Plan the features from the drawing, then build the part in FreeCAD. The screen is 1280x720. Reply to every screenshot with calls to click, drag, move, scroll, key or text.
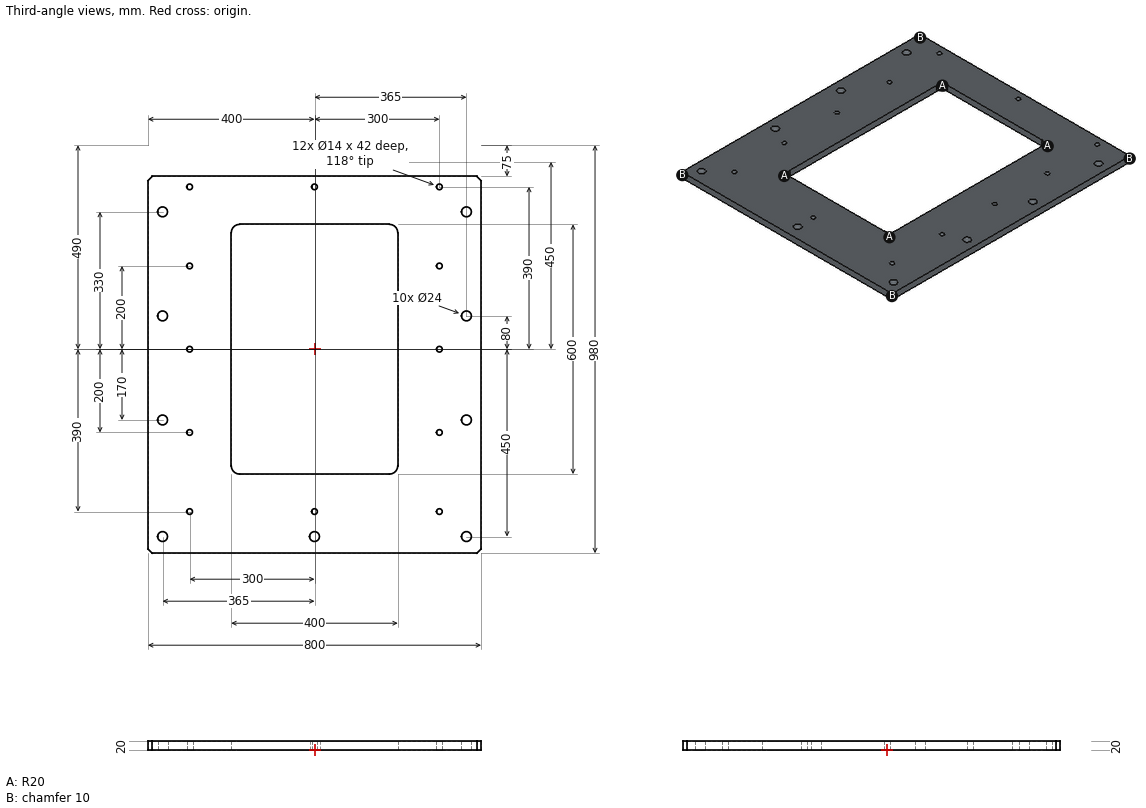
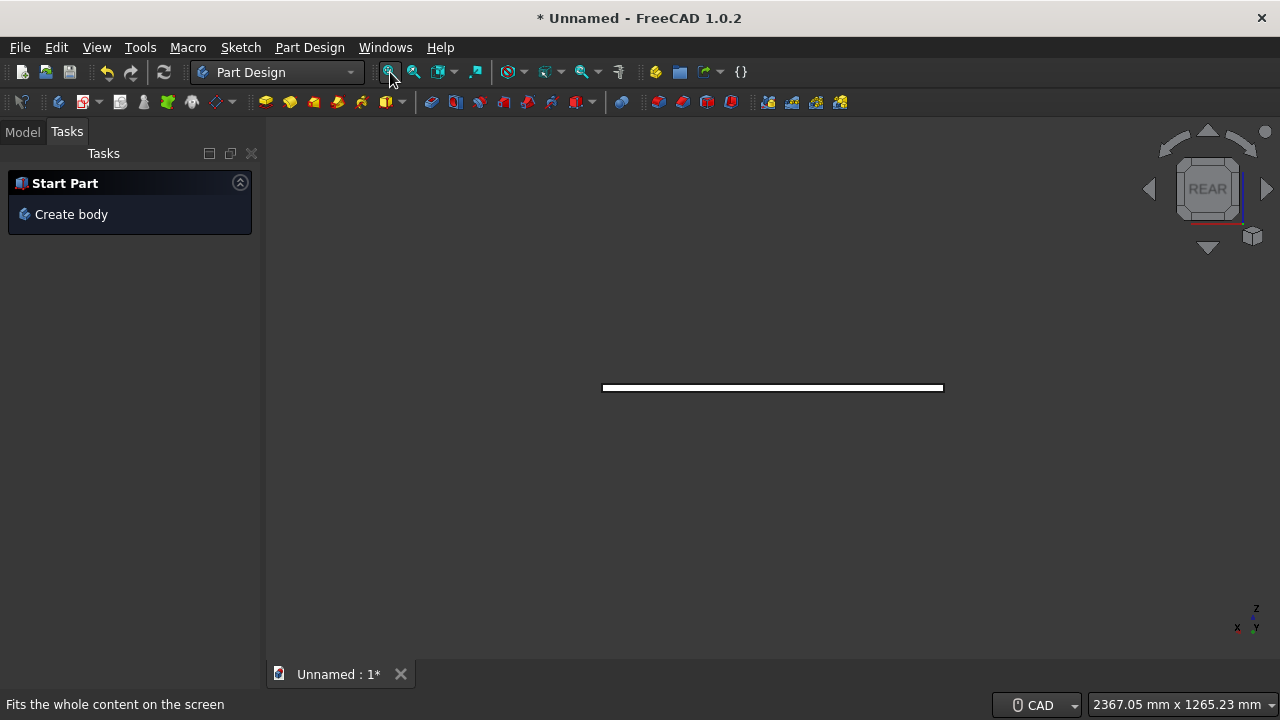
key(6)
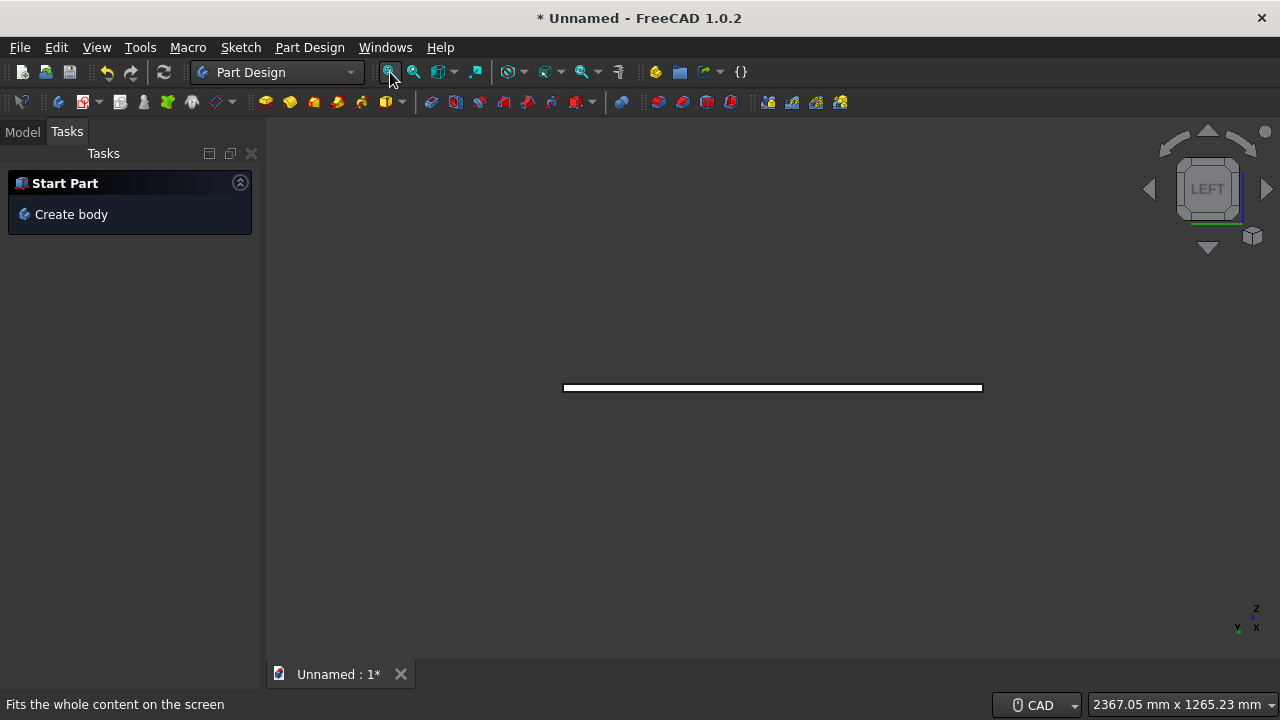
click(390, 72)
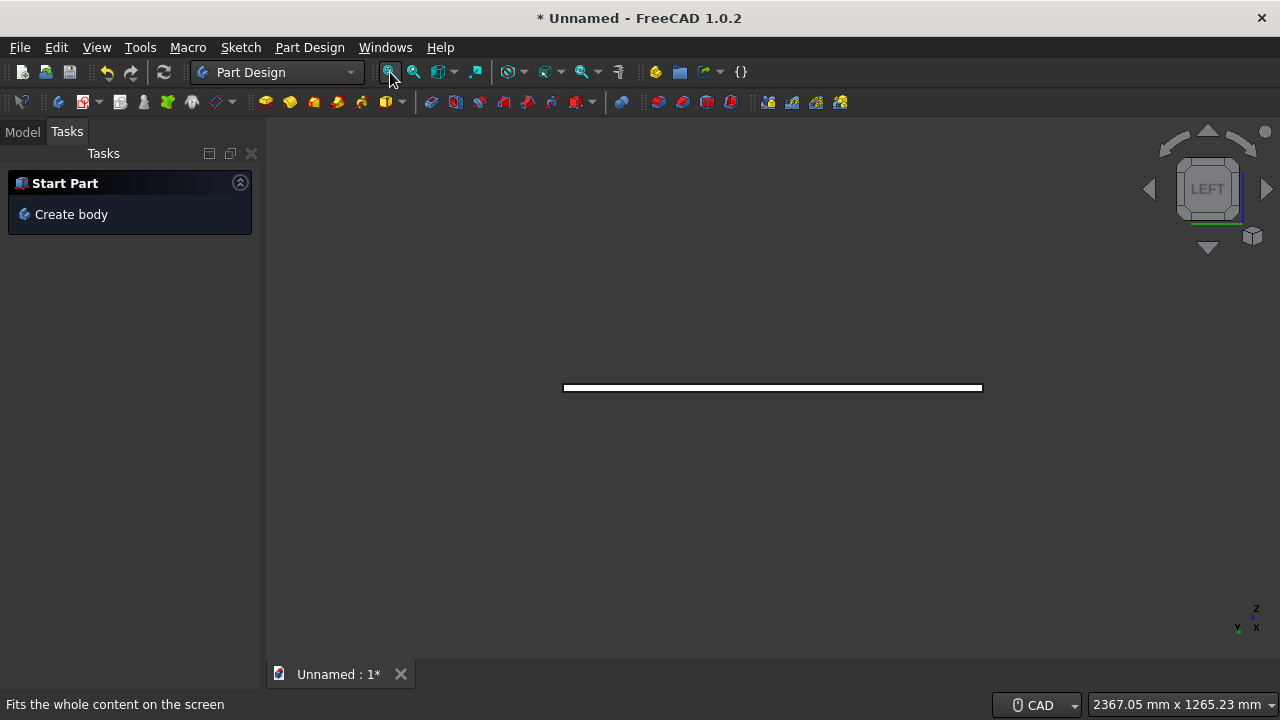
scroll(644, 387, up, 8)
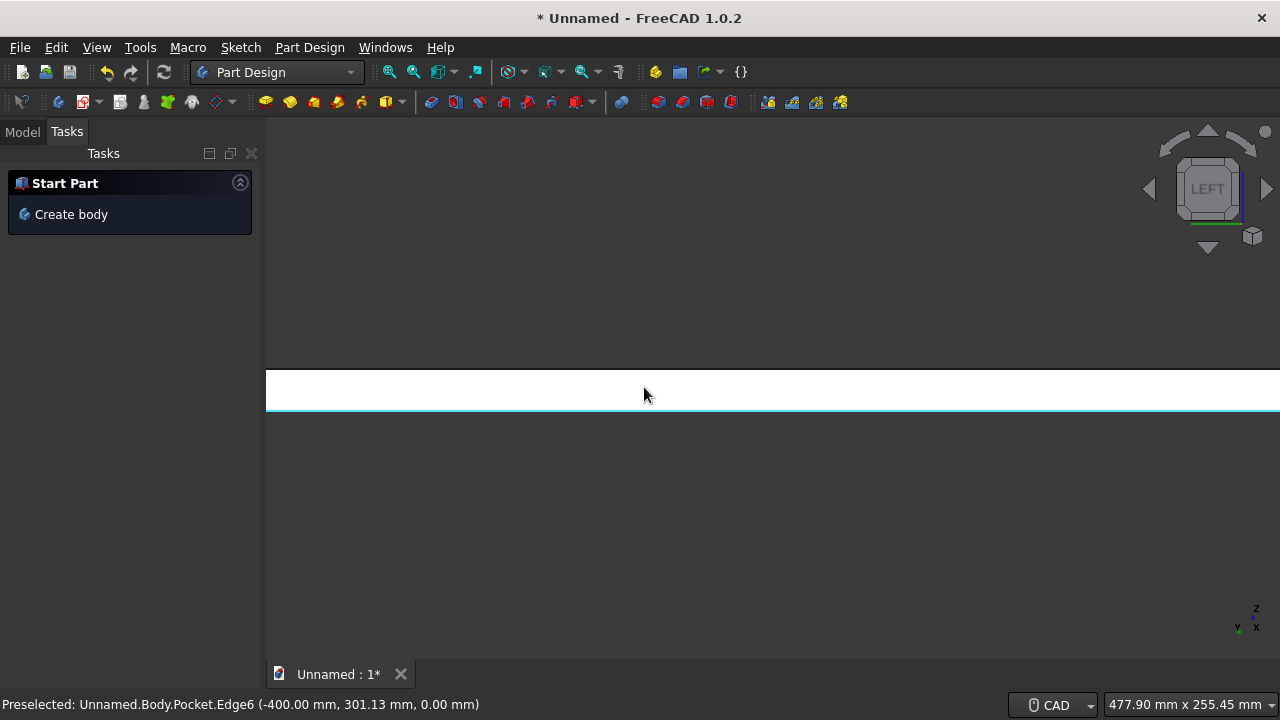
click(390, 72)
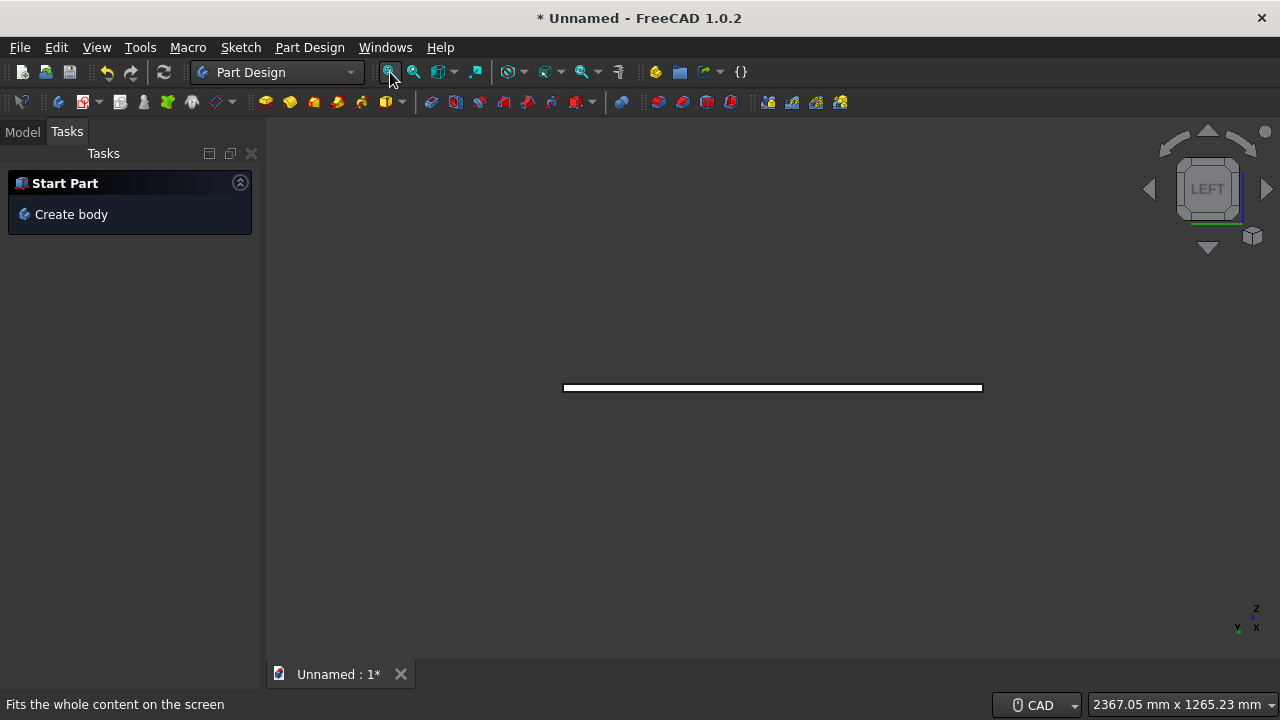
key(v)
key(3)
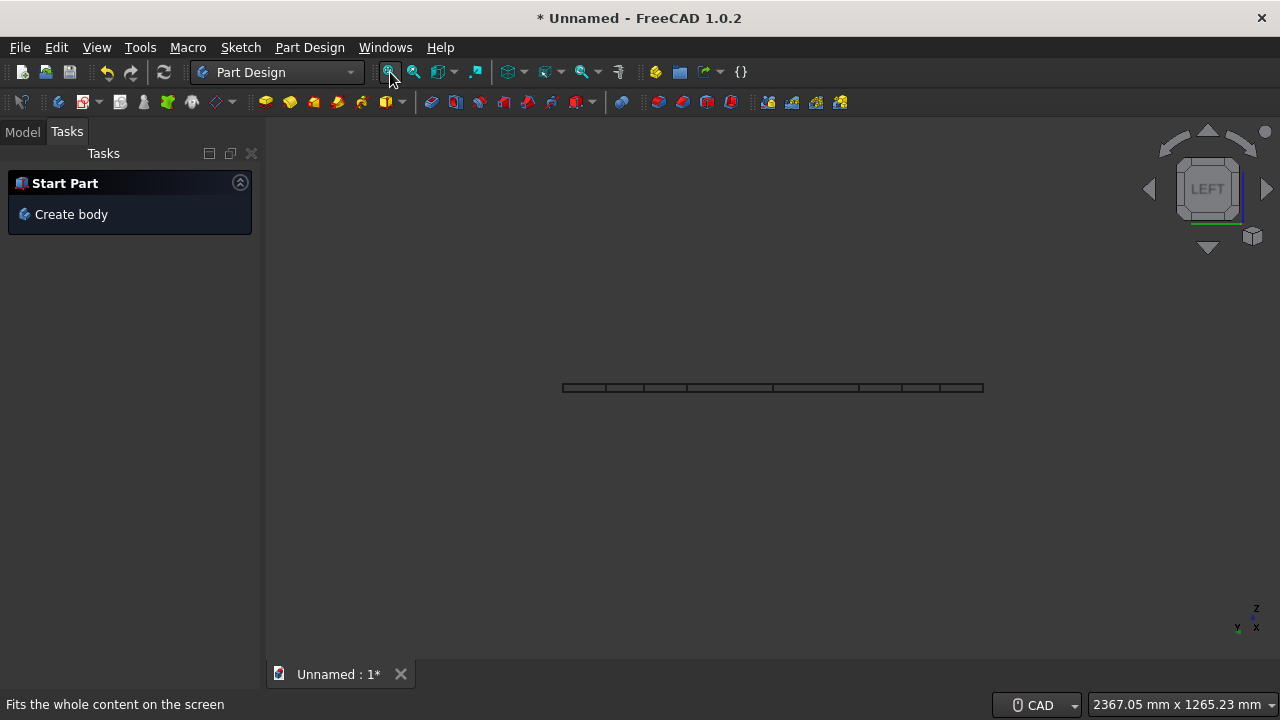
key(0)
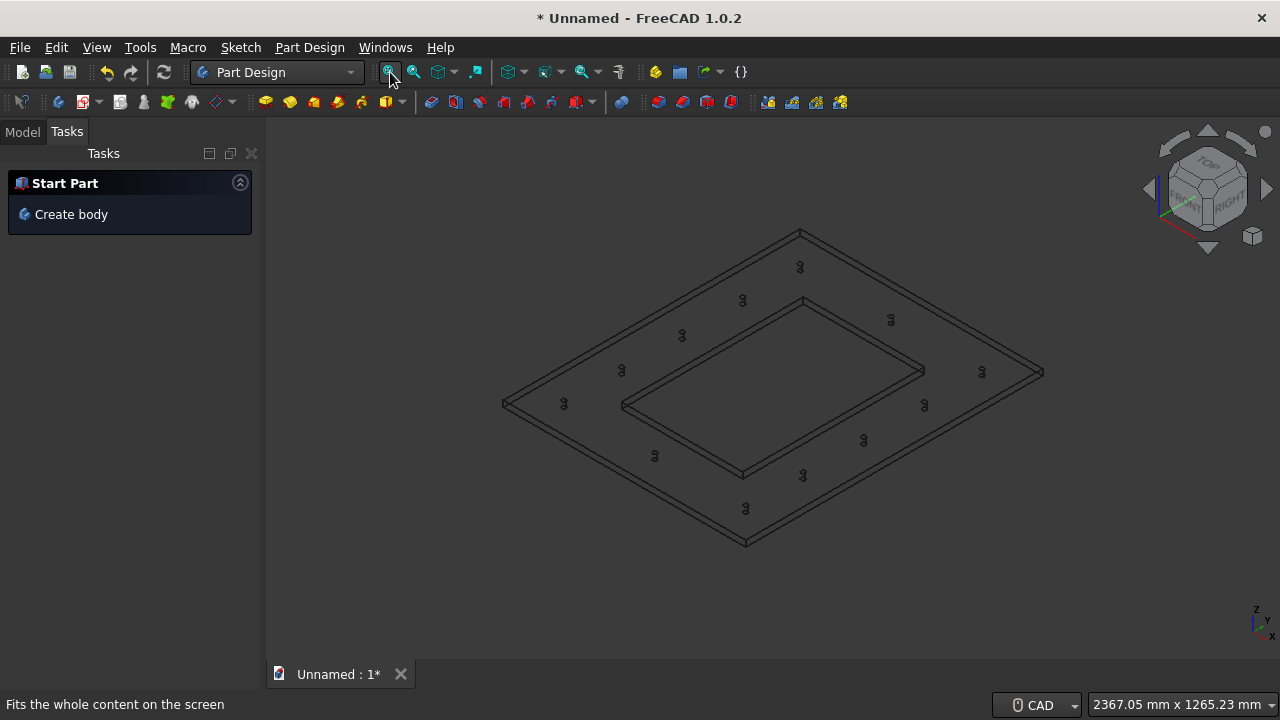
scroll(924, 370, up, 8)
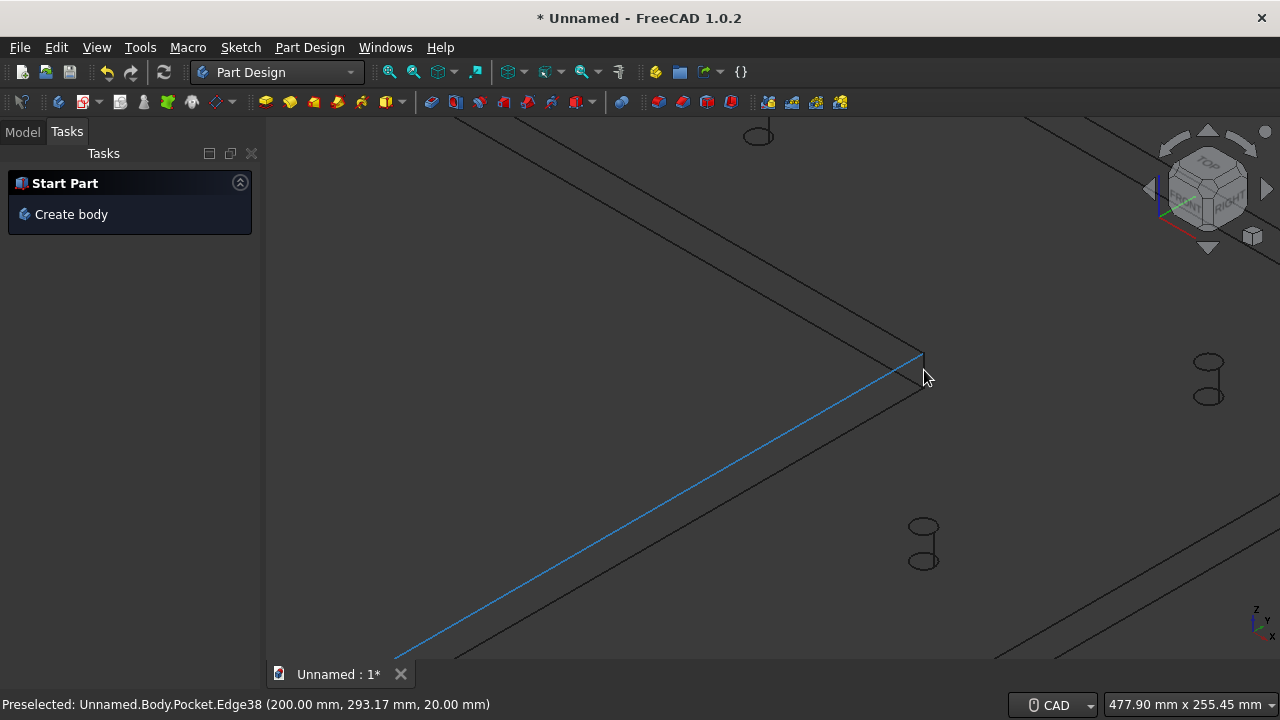
click(924, 370)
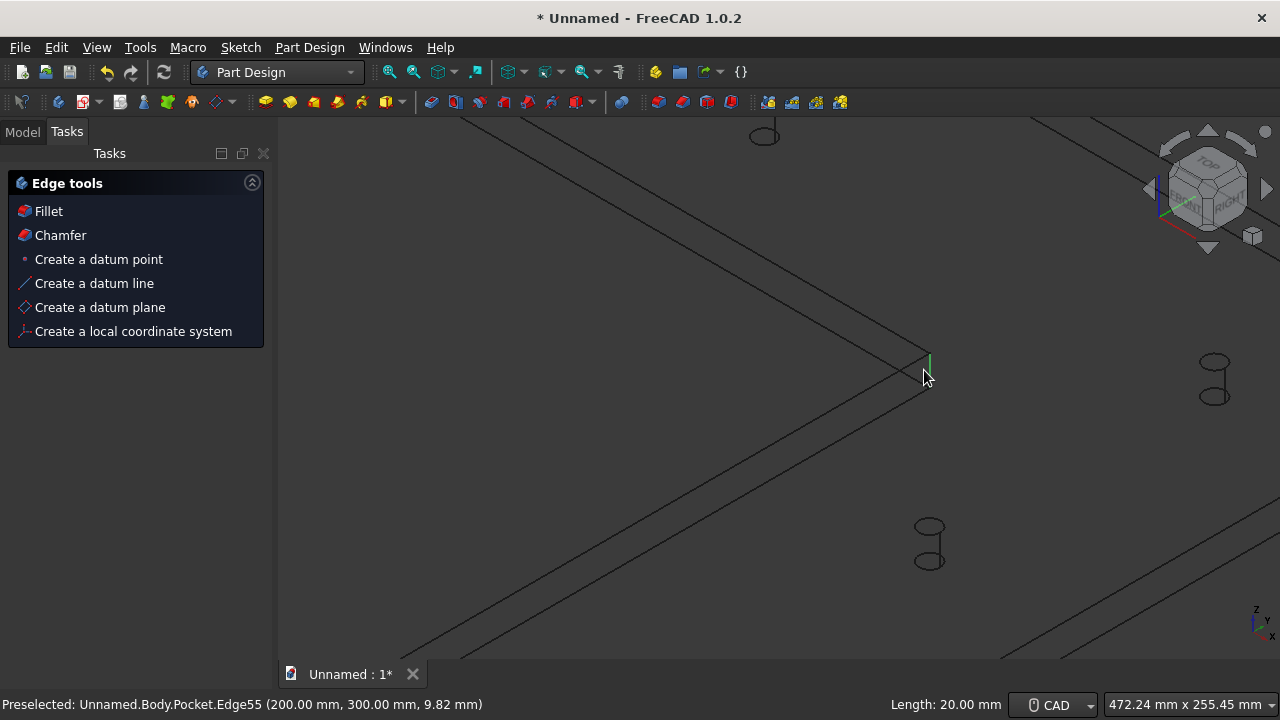
click(390, 72)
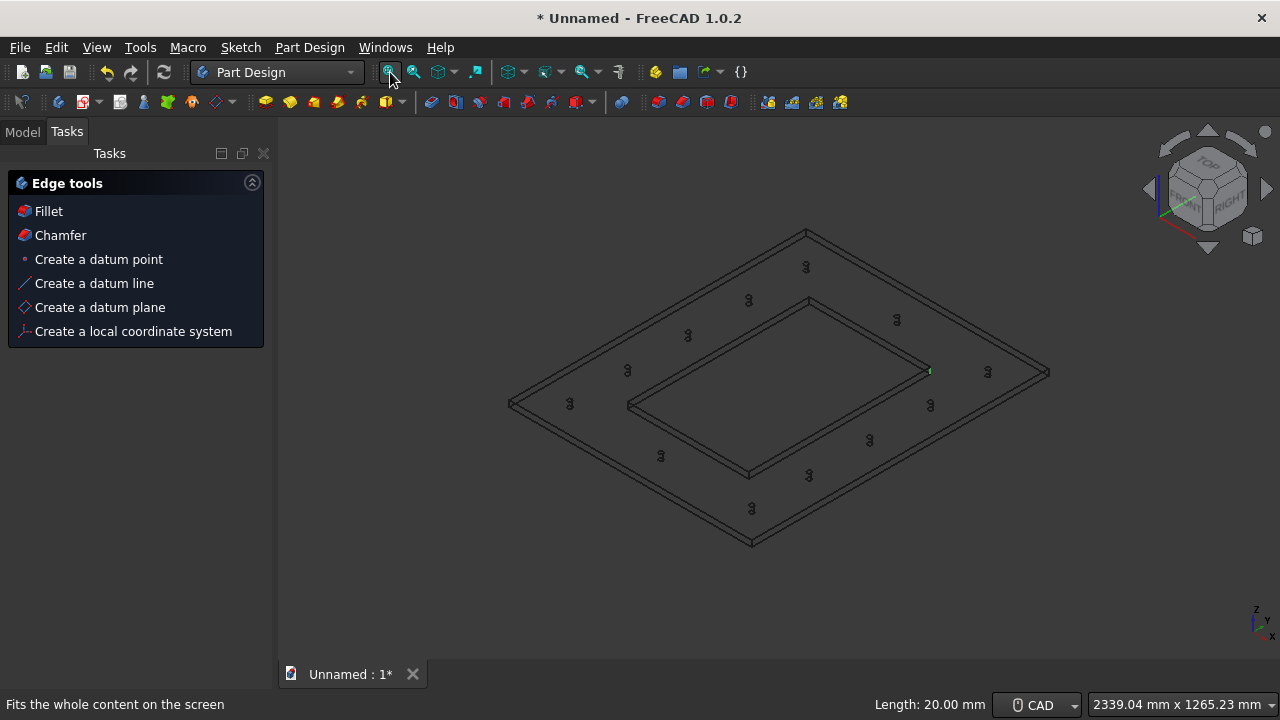
key(2)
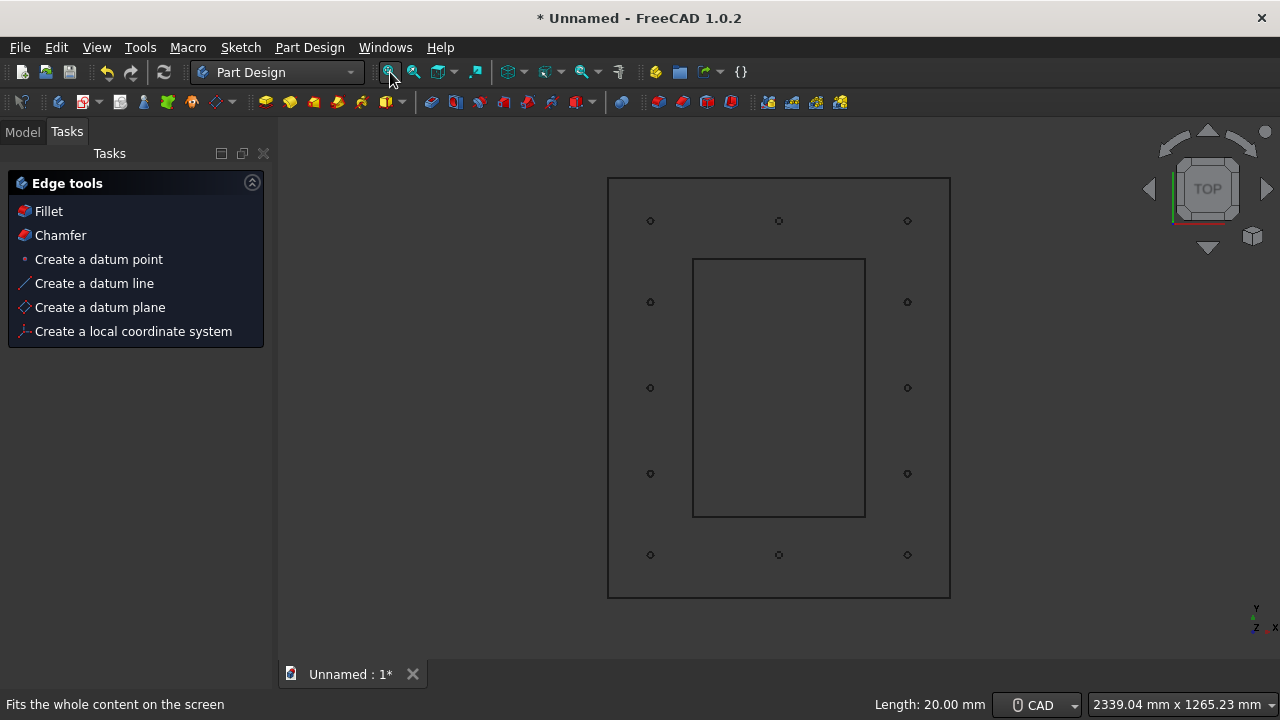
scroll(865, 516, up, 8)